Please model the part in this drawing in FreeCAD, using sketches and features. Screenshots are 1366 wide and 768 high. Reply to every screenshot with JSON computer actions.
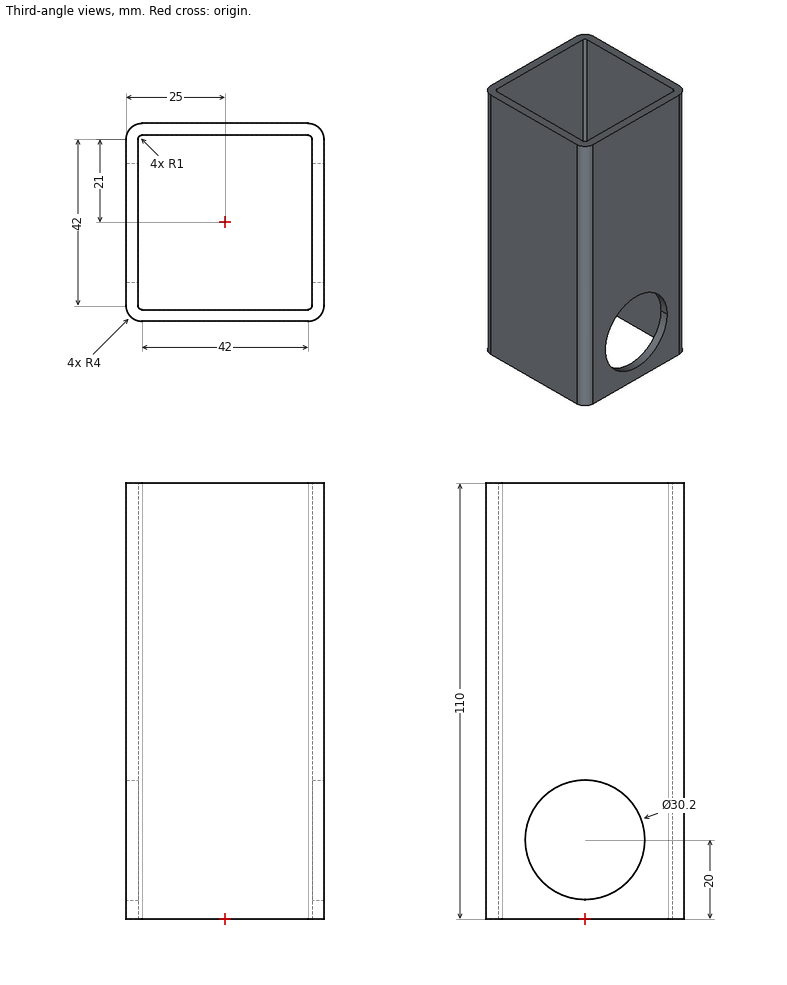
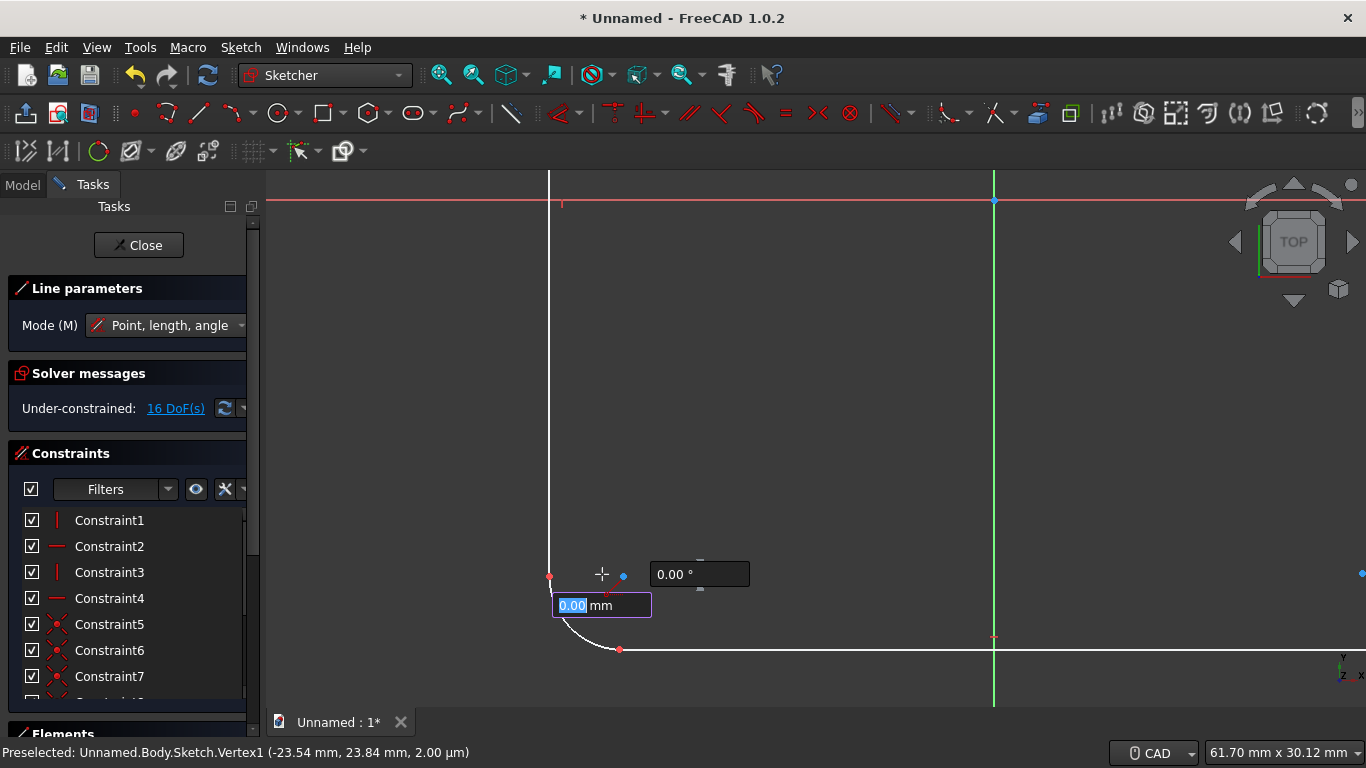
{"action": "scroll", "coordinate": [604, 577], "scroll_direction": "down", "scroll_amount": 5}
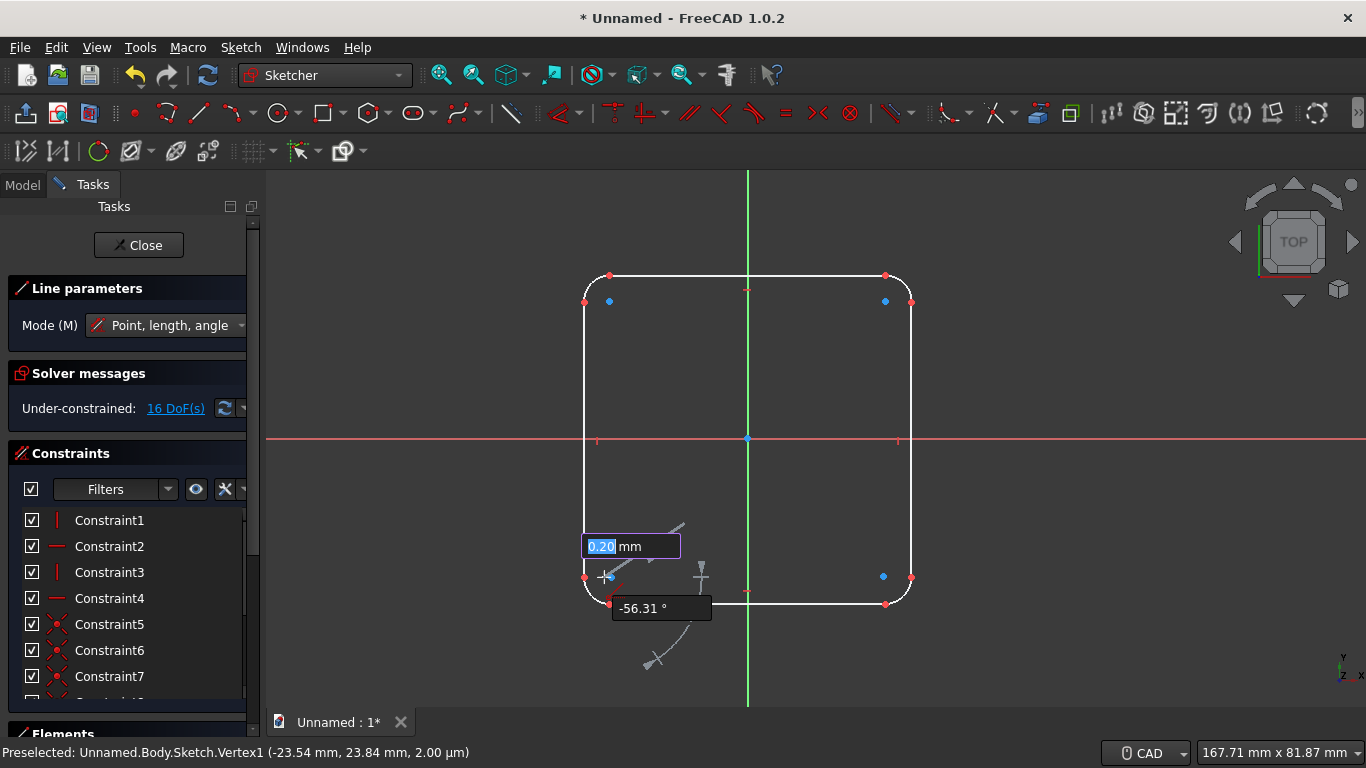
{"action": "scroll", "coordinate": [604, 301], "scroll_direction": "up", "scroll_amount": 5}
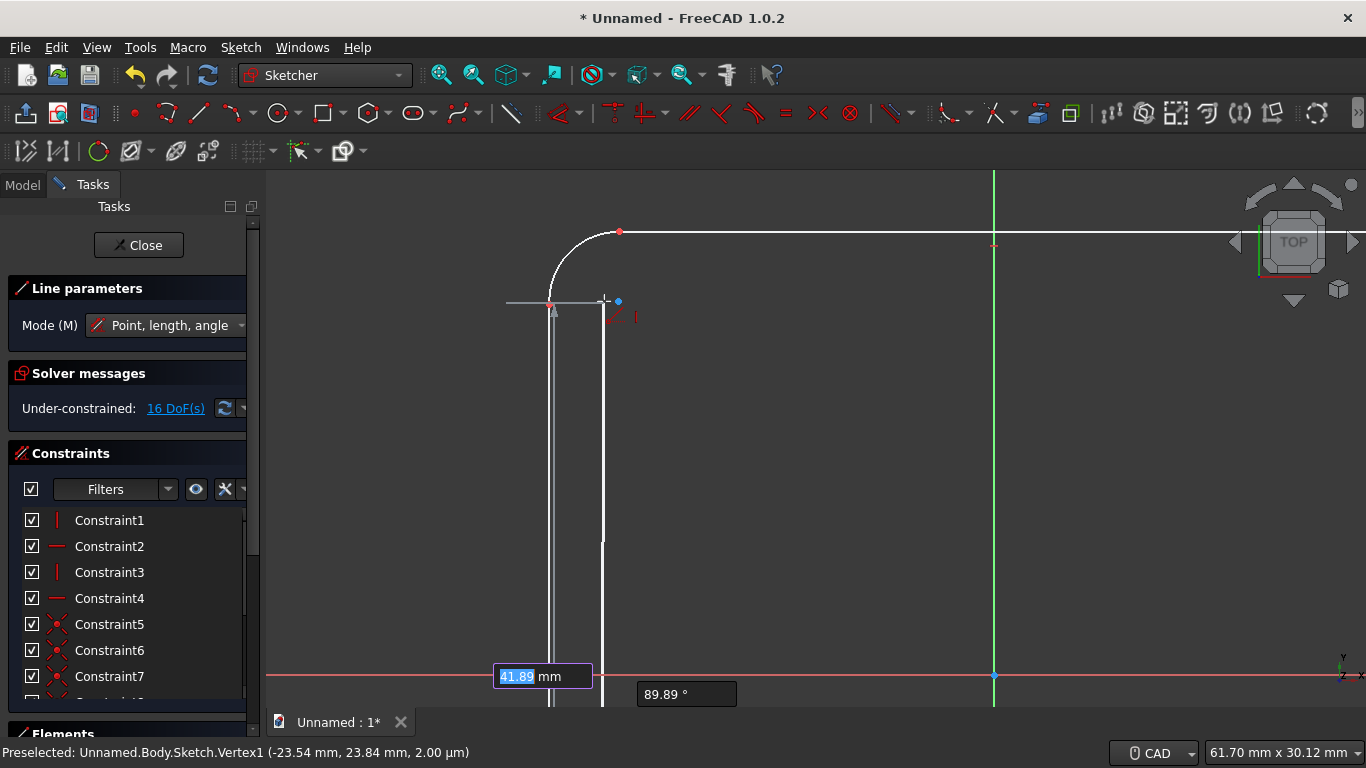
{"action": "left_click", "coordinate": [602, 301]}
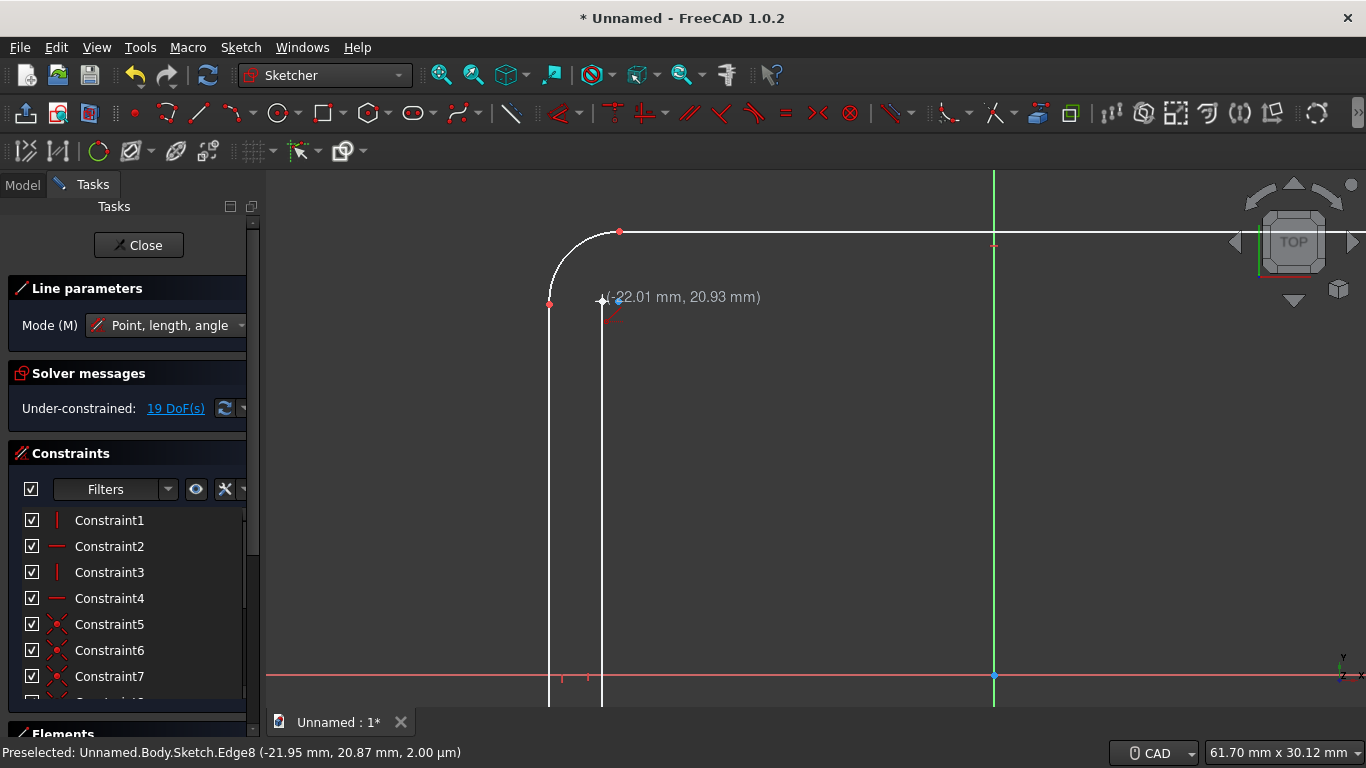
{"action": "left_click", "coordinate": [620, 283]}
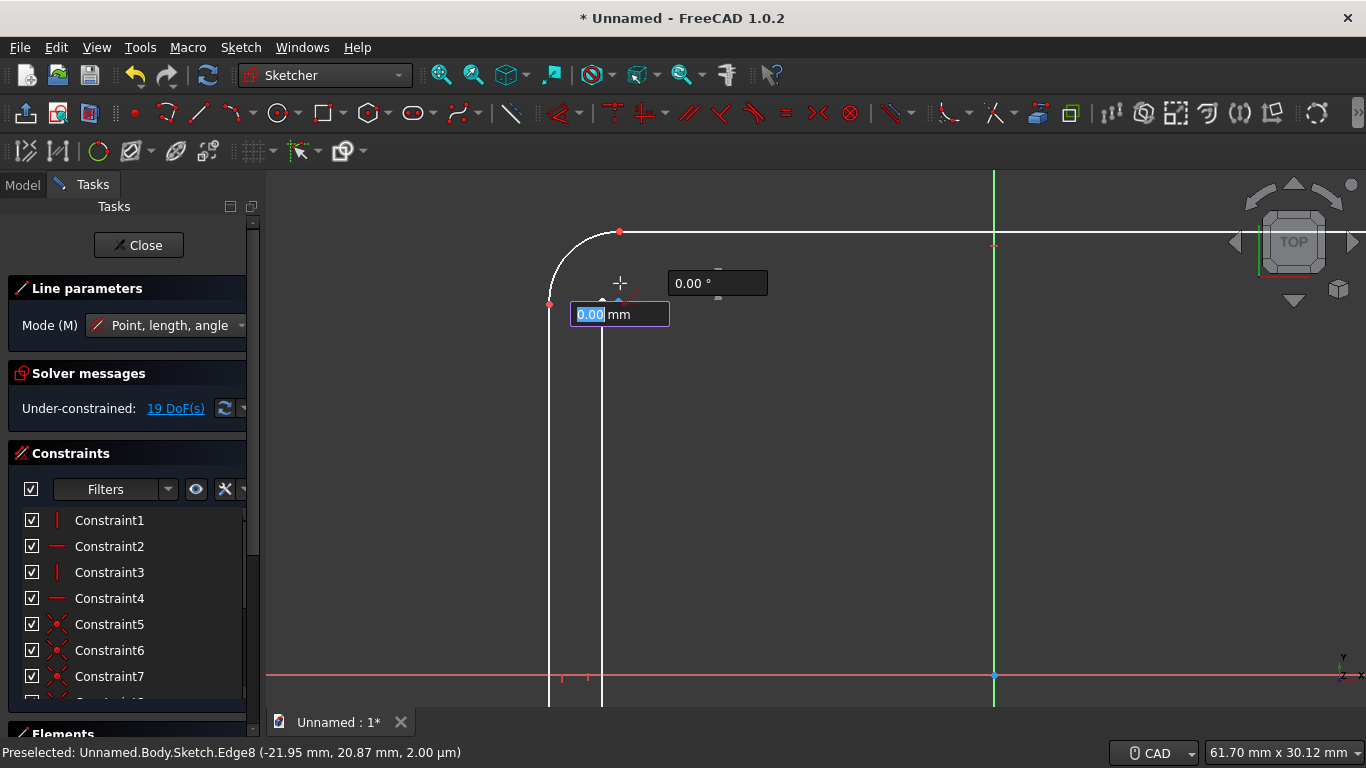
{"action": "scroll", "coordinate": [604, 301], "scroll_direction": "down", "scroll_amount": 5}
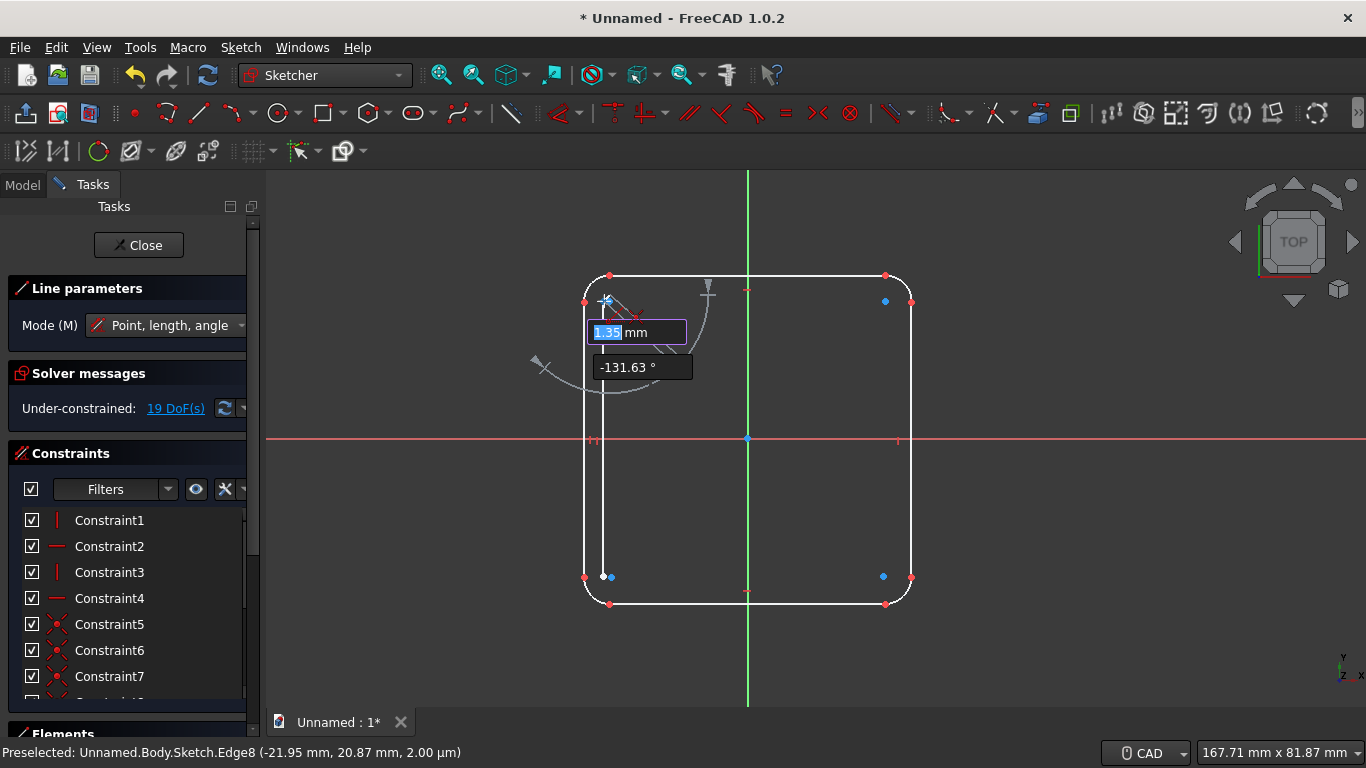
{"action": "scroll", "coordinate": [886, 294], "scroll_direction": "up", "scroll_amount": 5}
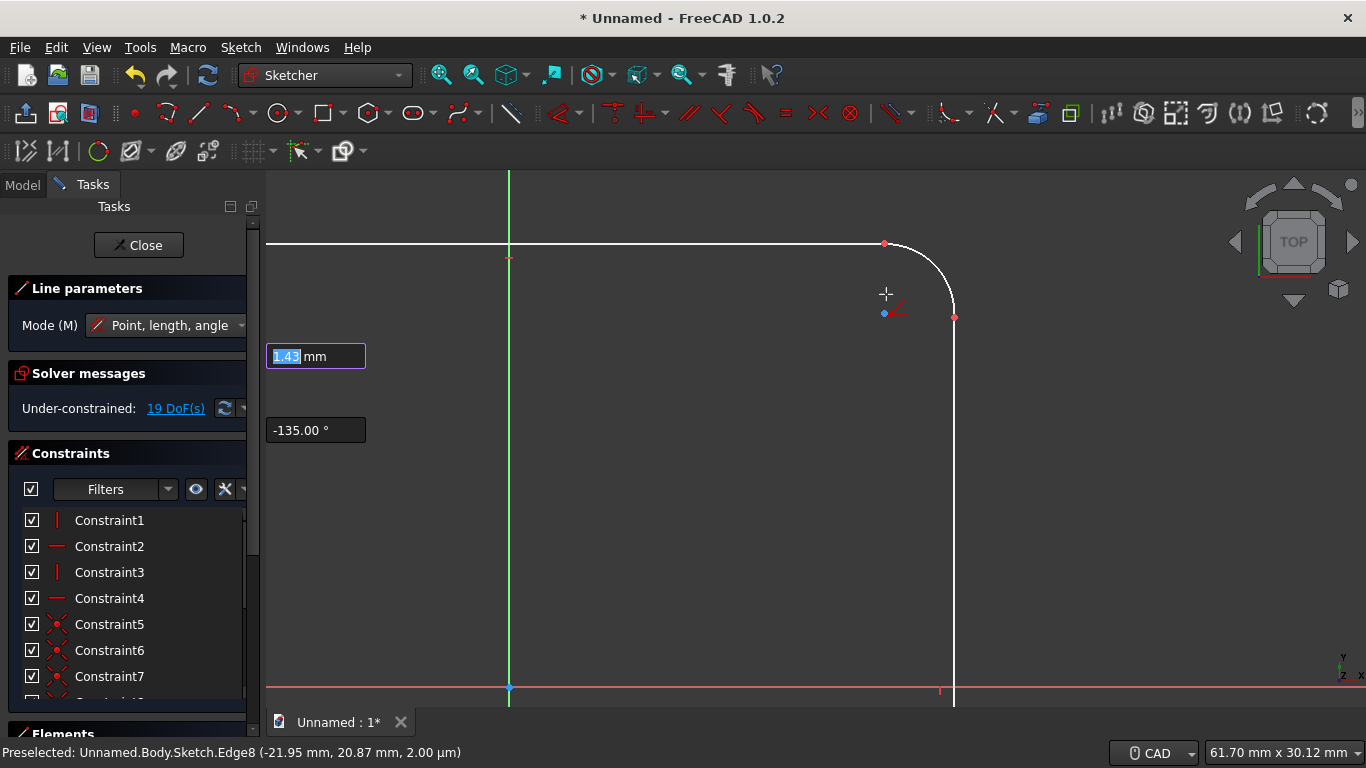
{"action": "left_click", "coordinate": [884, 295]}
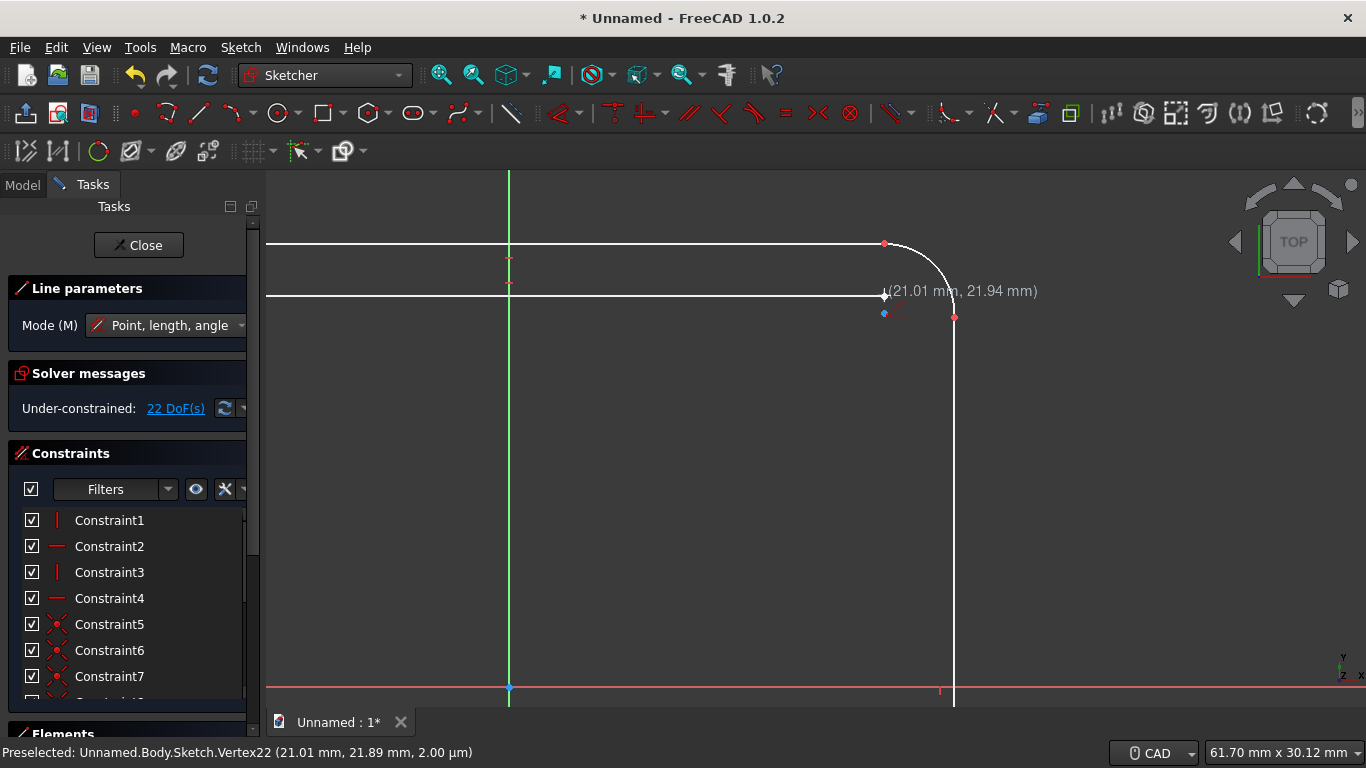
{"action": "left_click", "coordinate": [902, 313]}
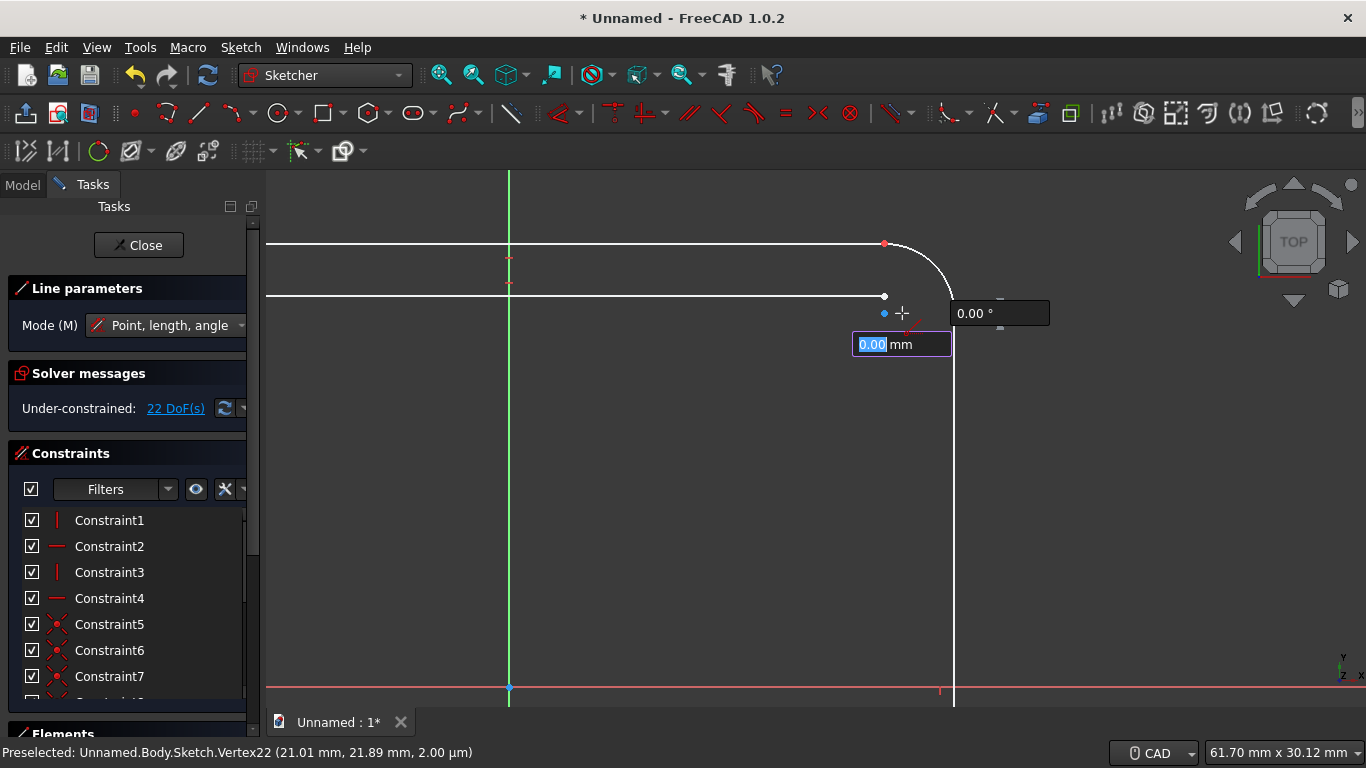
{"action": "scroll", "coordinate": [886, 294], "scroll_direction": "down", "scroll_amount": 5}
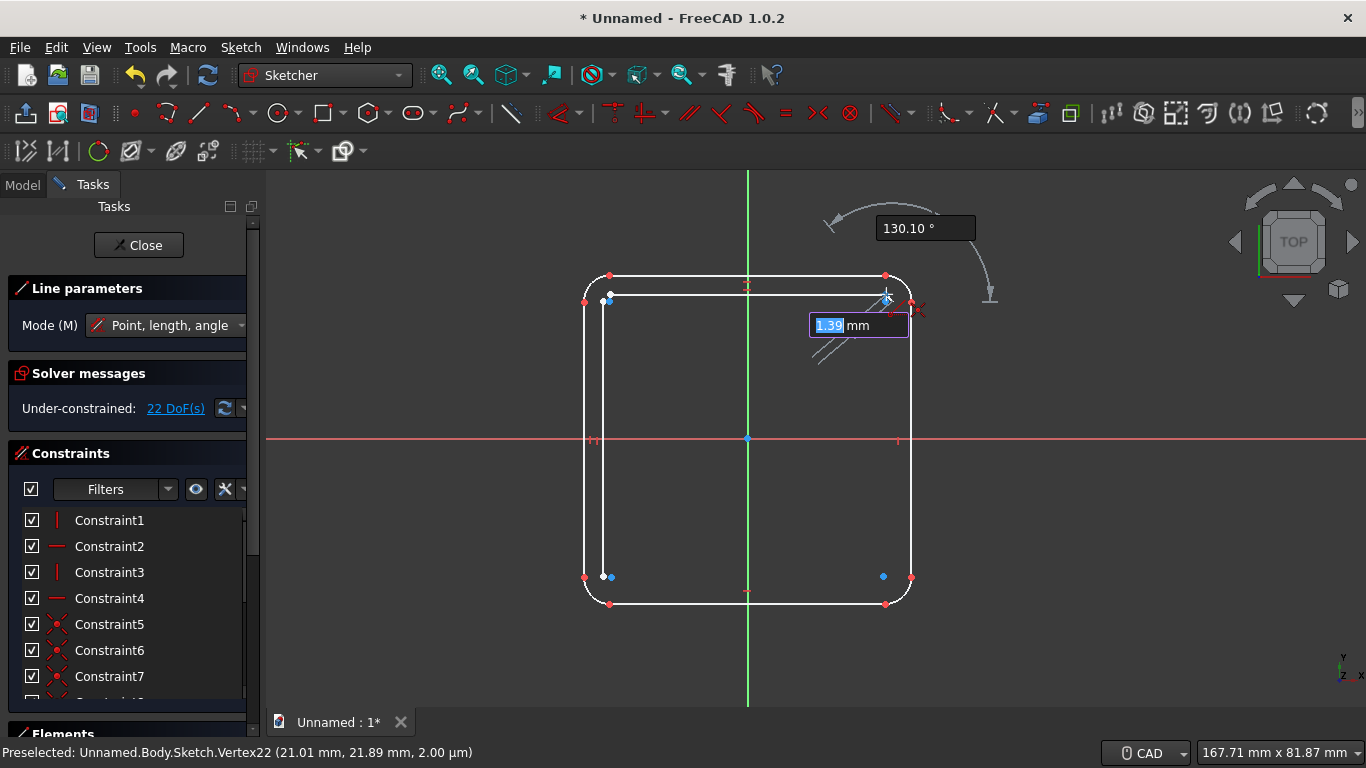
{"action": "scroll", "coordinate": [892, 577], "scroll_direction": "up", "scroll_amount": 5}